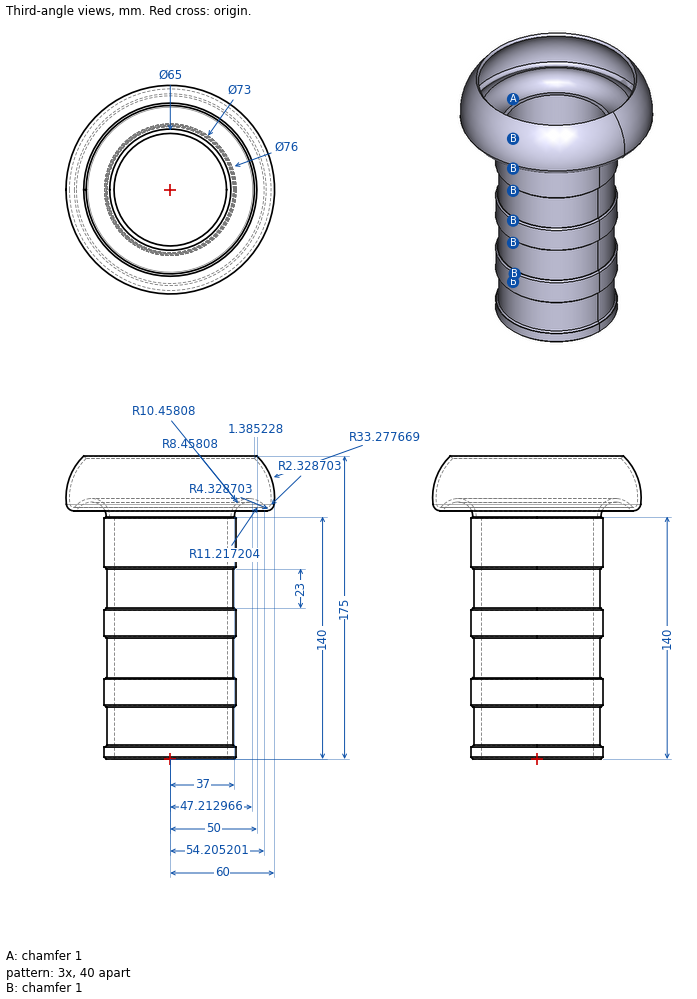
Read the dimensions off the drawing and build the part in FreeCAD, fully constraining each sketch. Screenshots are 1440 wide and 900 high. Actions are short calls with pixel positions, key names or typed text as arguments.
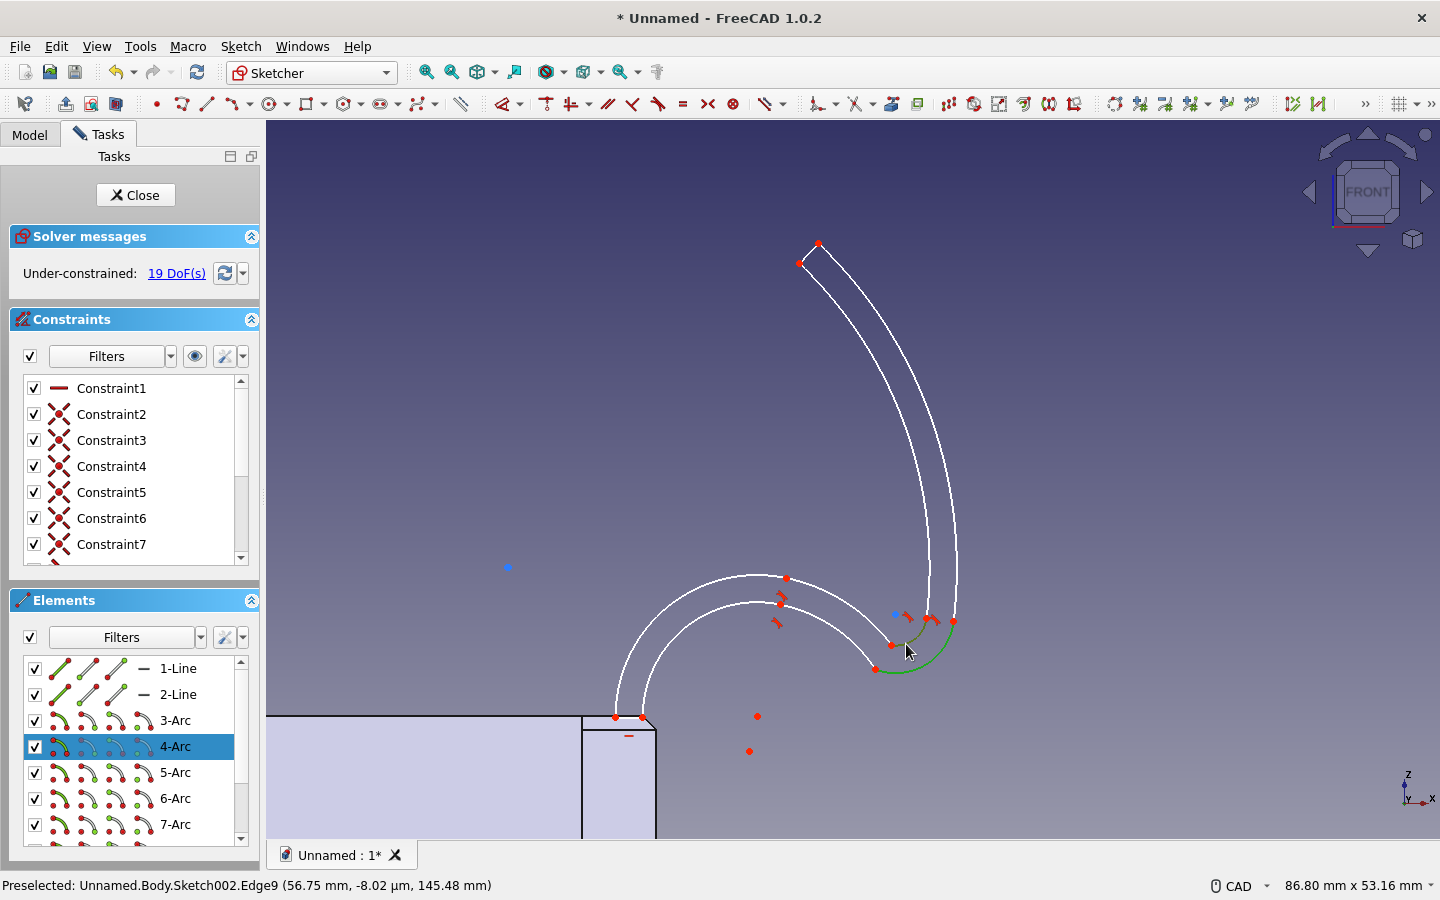
click(546, 104)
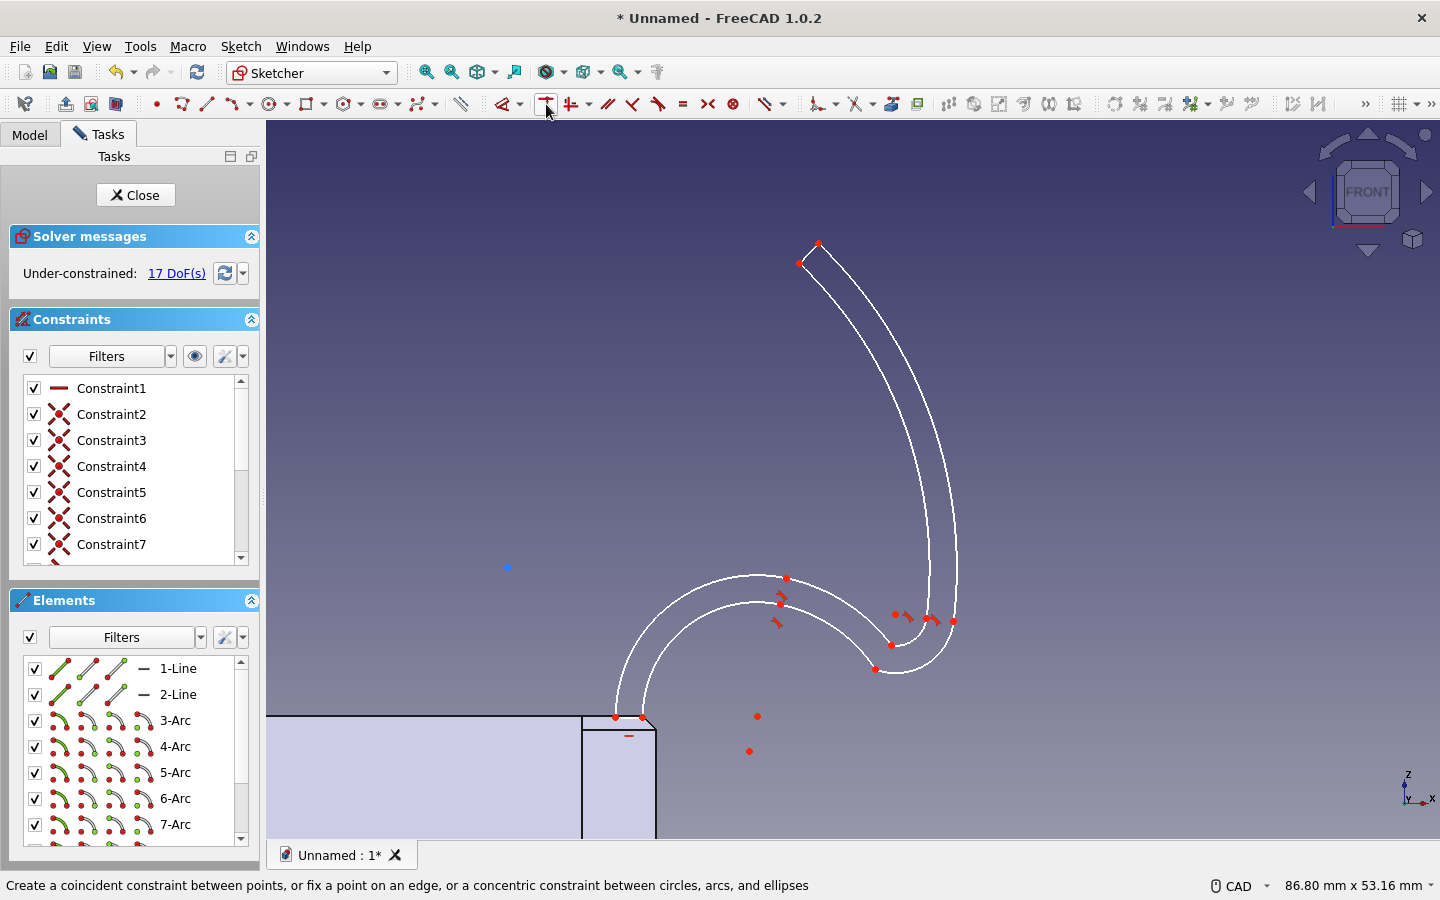
click(951, 497)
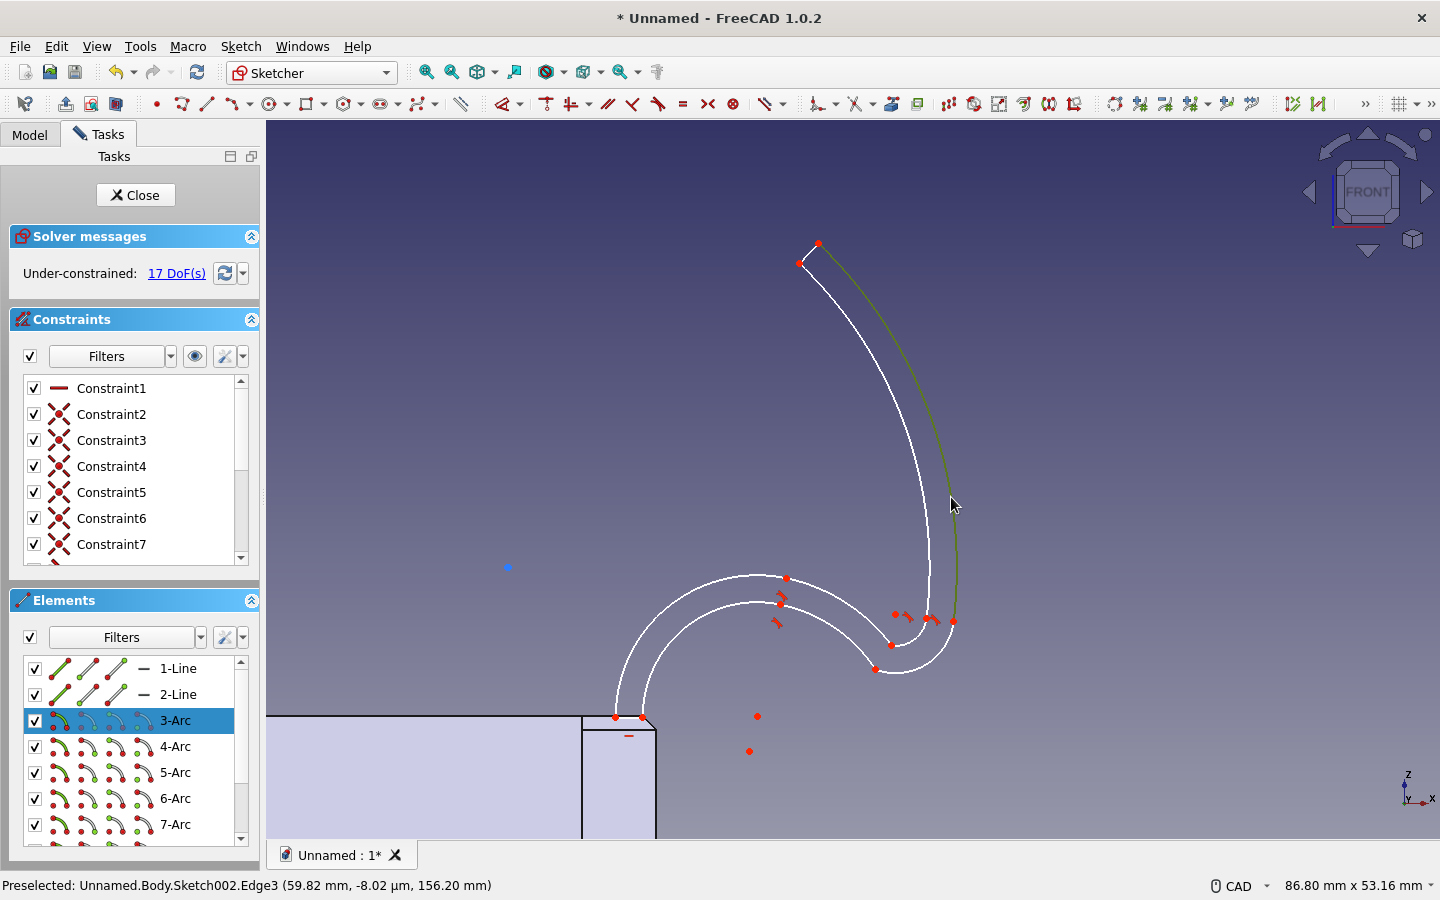
click(924, 502)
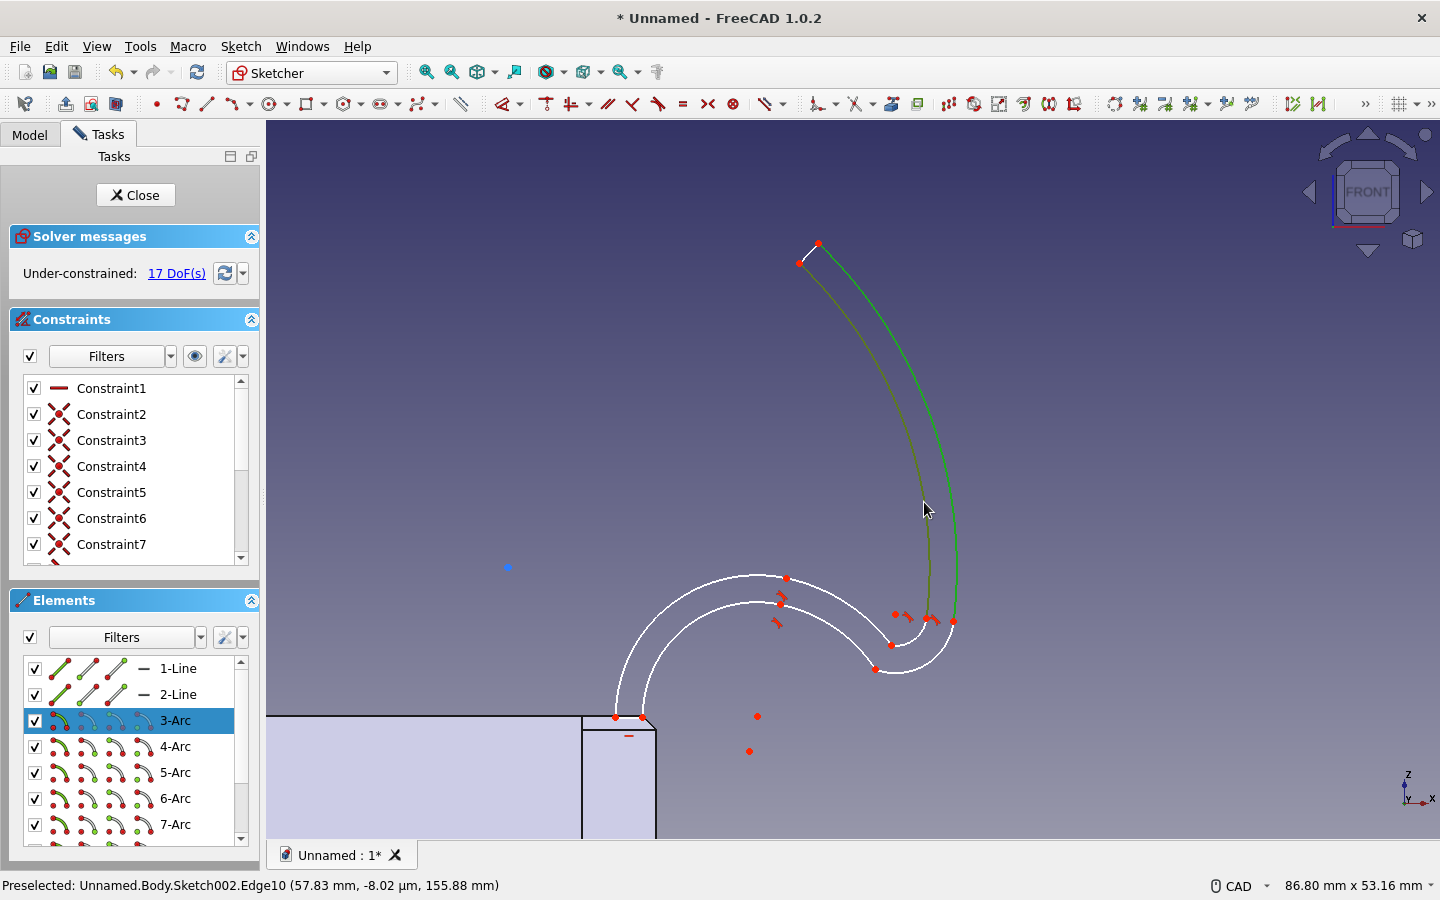
click(546, 104)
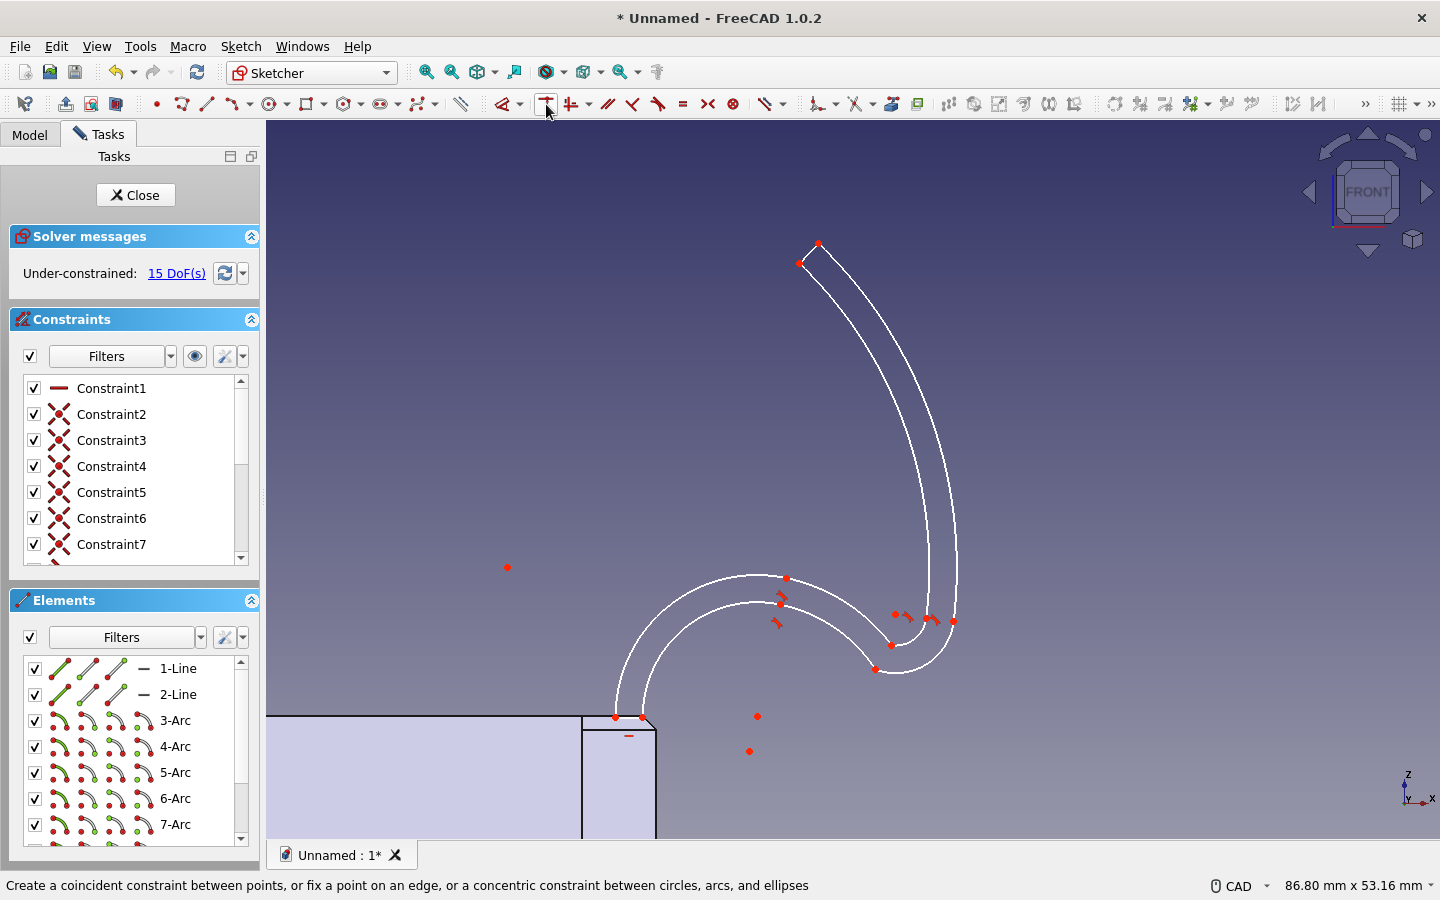
click(502, 104)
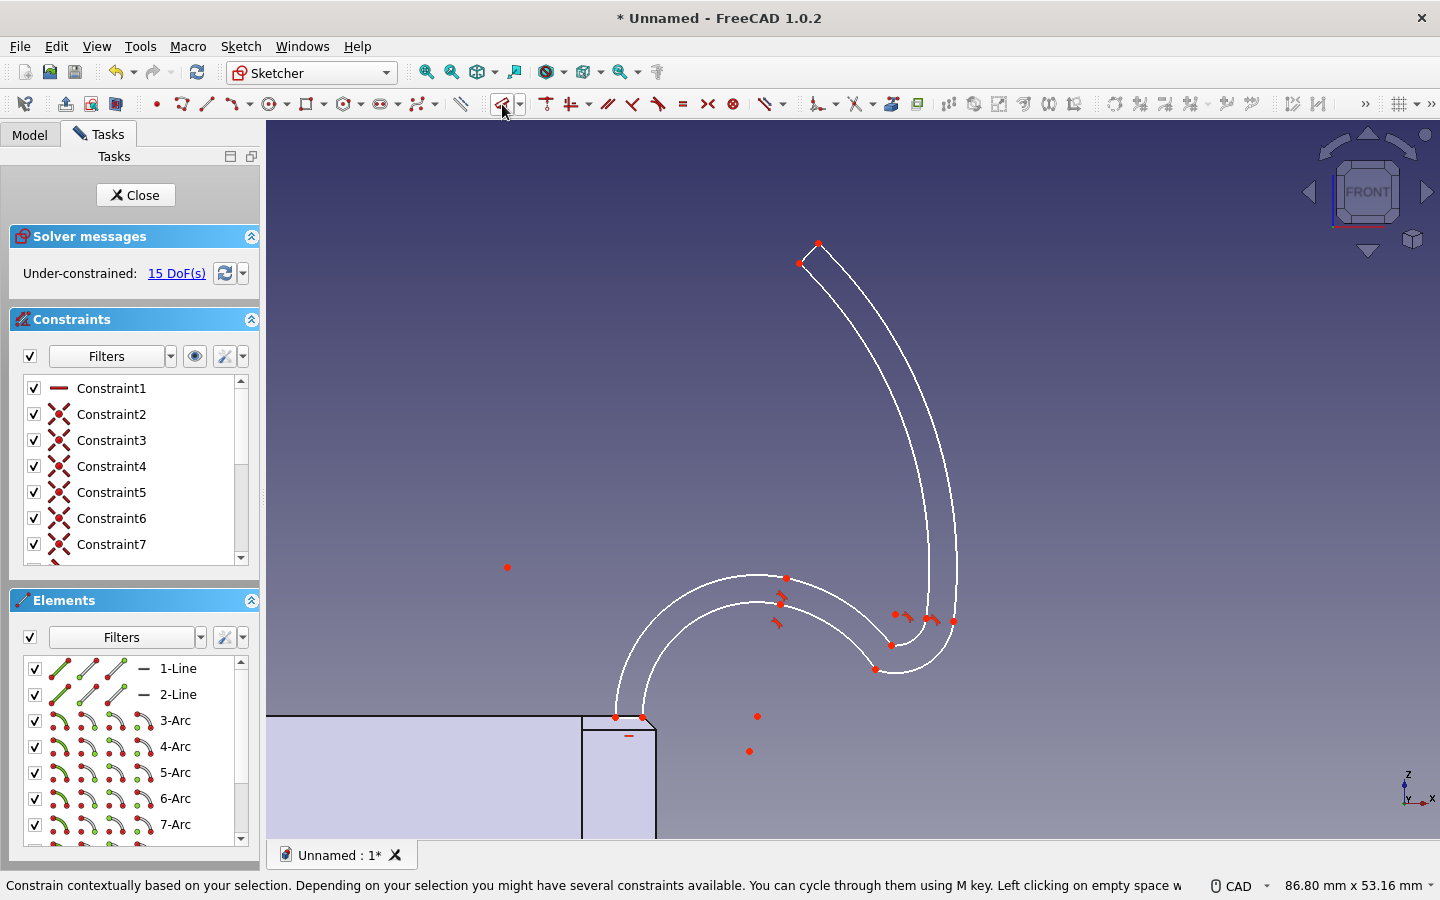
click(951, 497)
click(983, 492)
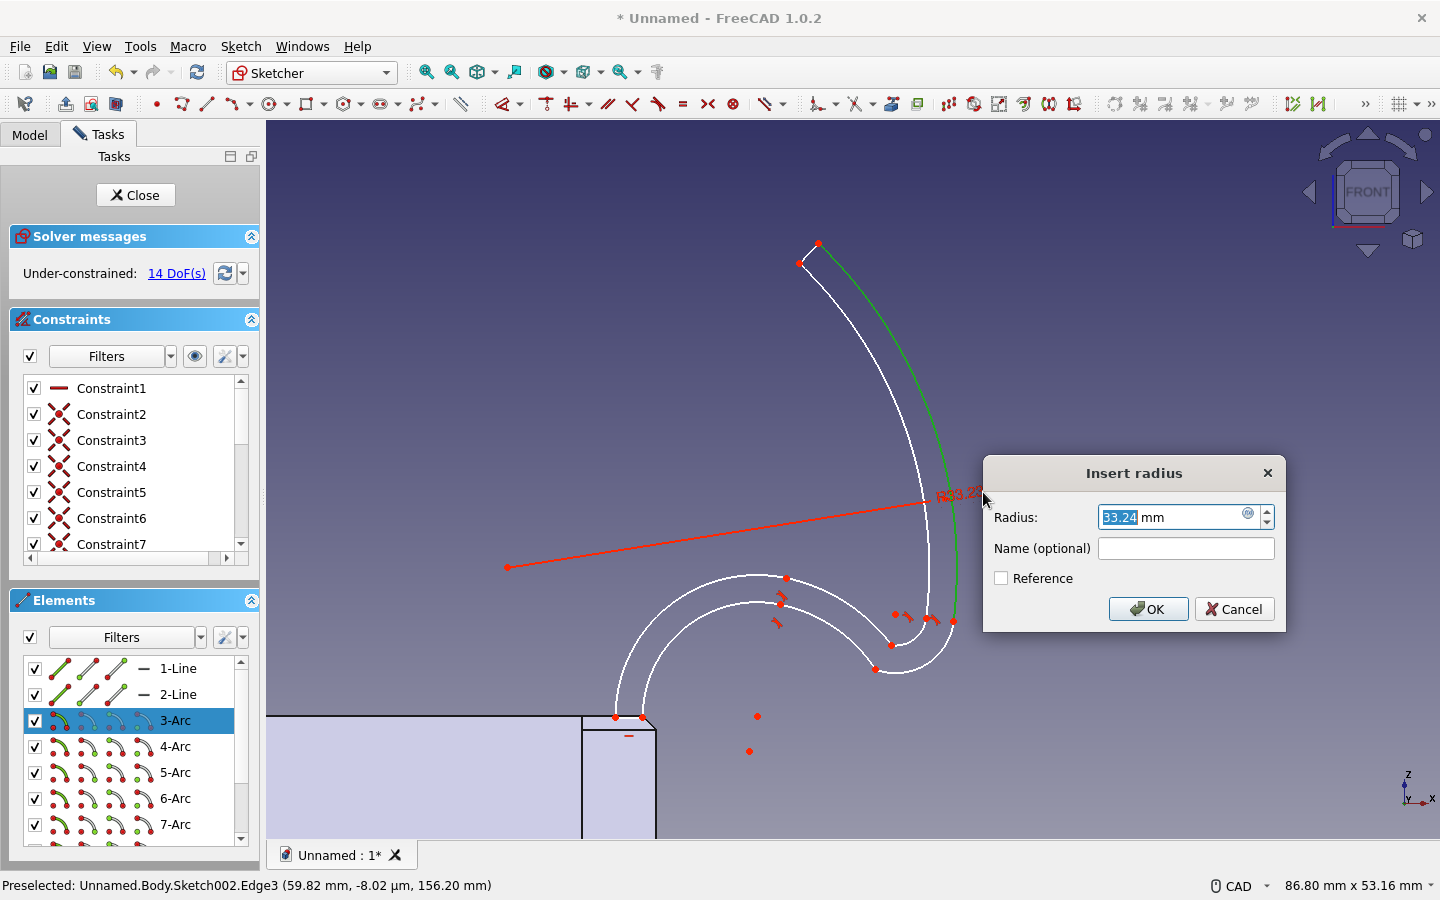
text(33.277669)
key(Return)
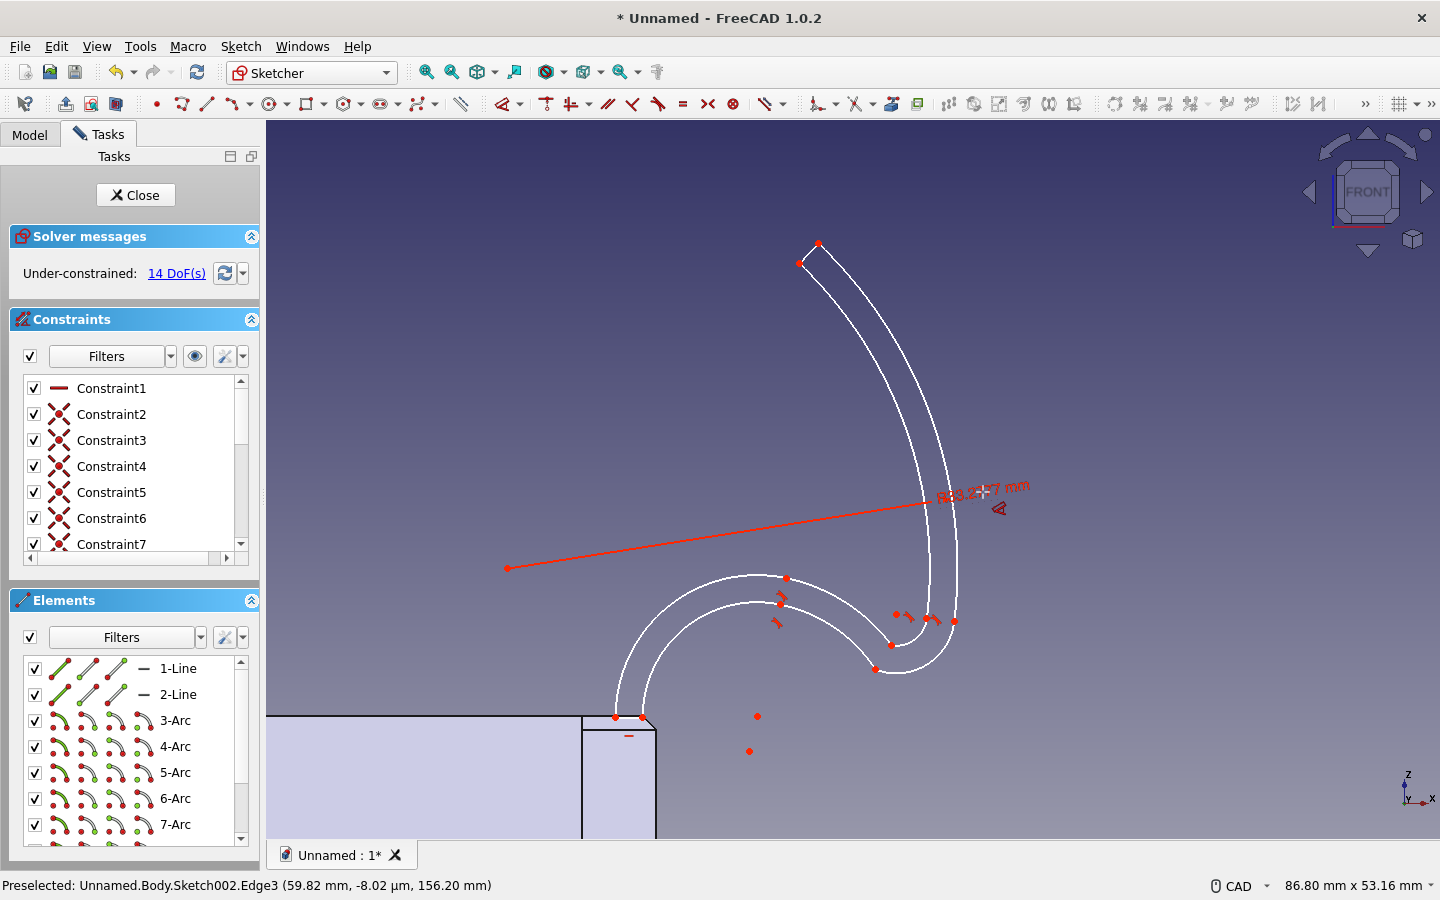
click(907, 672)
click(913, 703)